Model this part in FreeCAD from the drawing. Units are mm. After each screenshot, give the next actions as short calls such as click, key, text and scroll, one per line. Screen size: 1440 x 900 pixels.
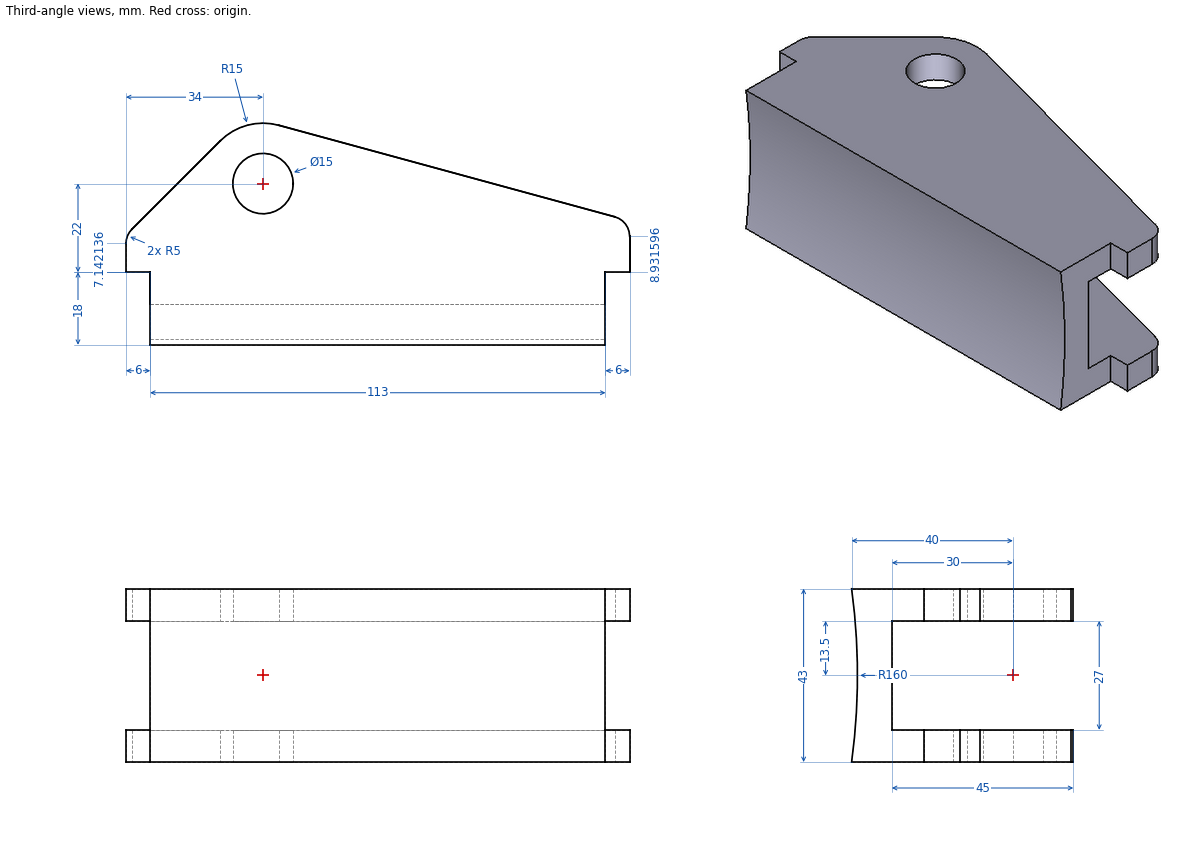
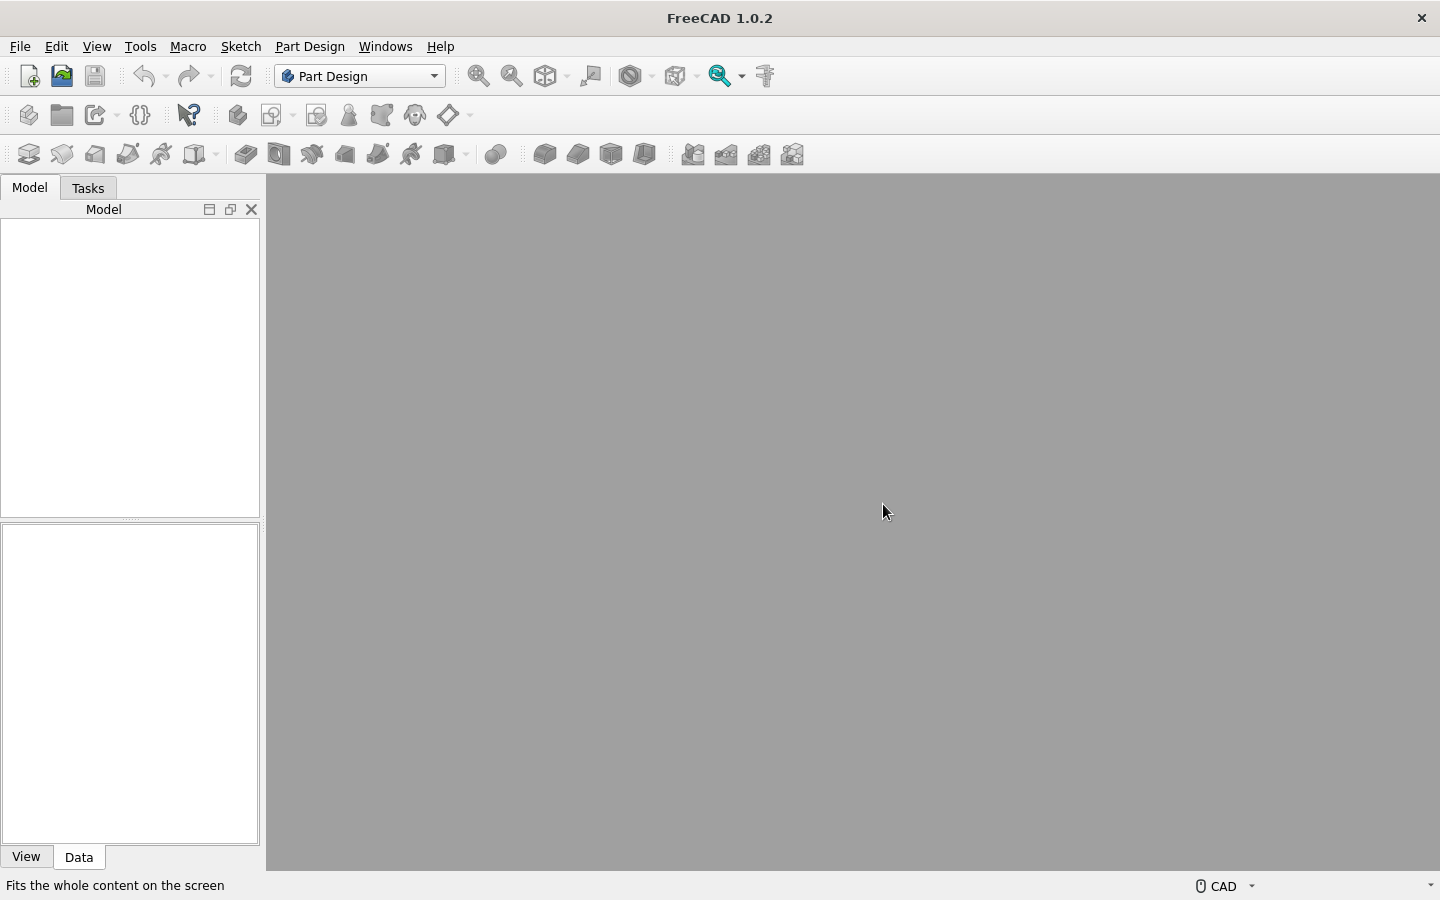
click(29, 76)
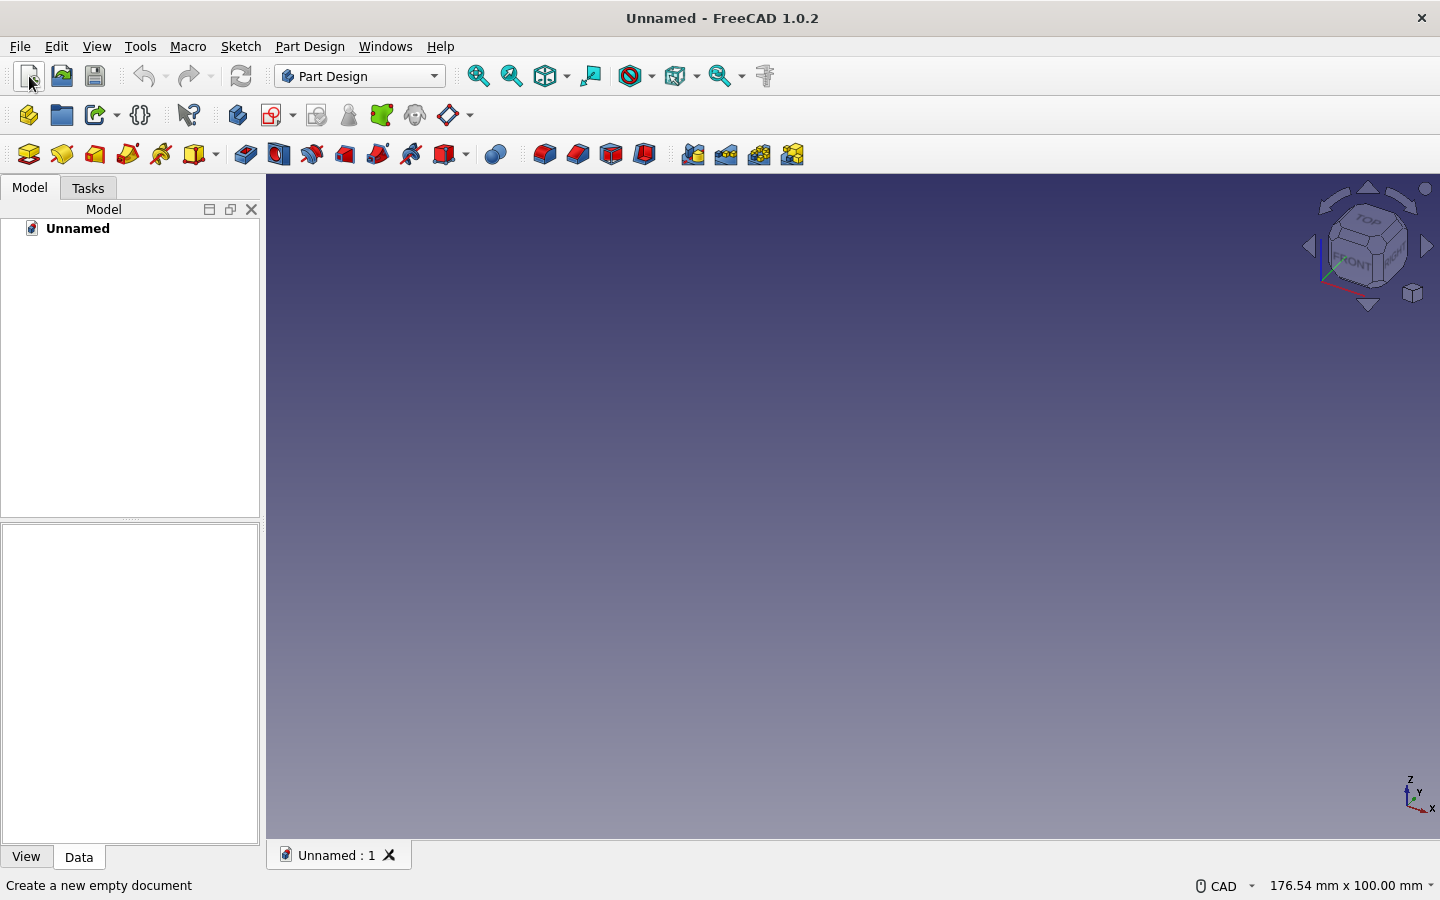
click(270, 116)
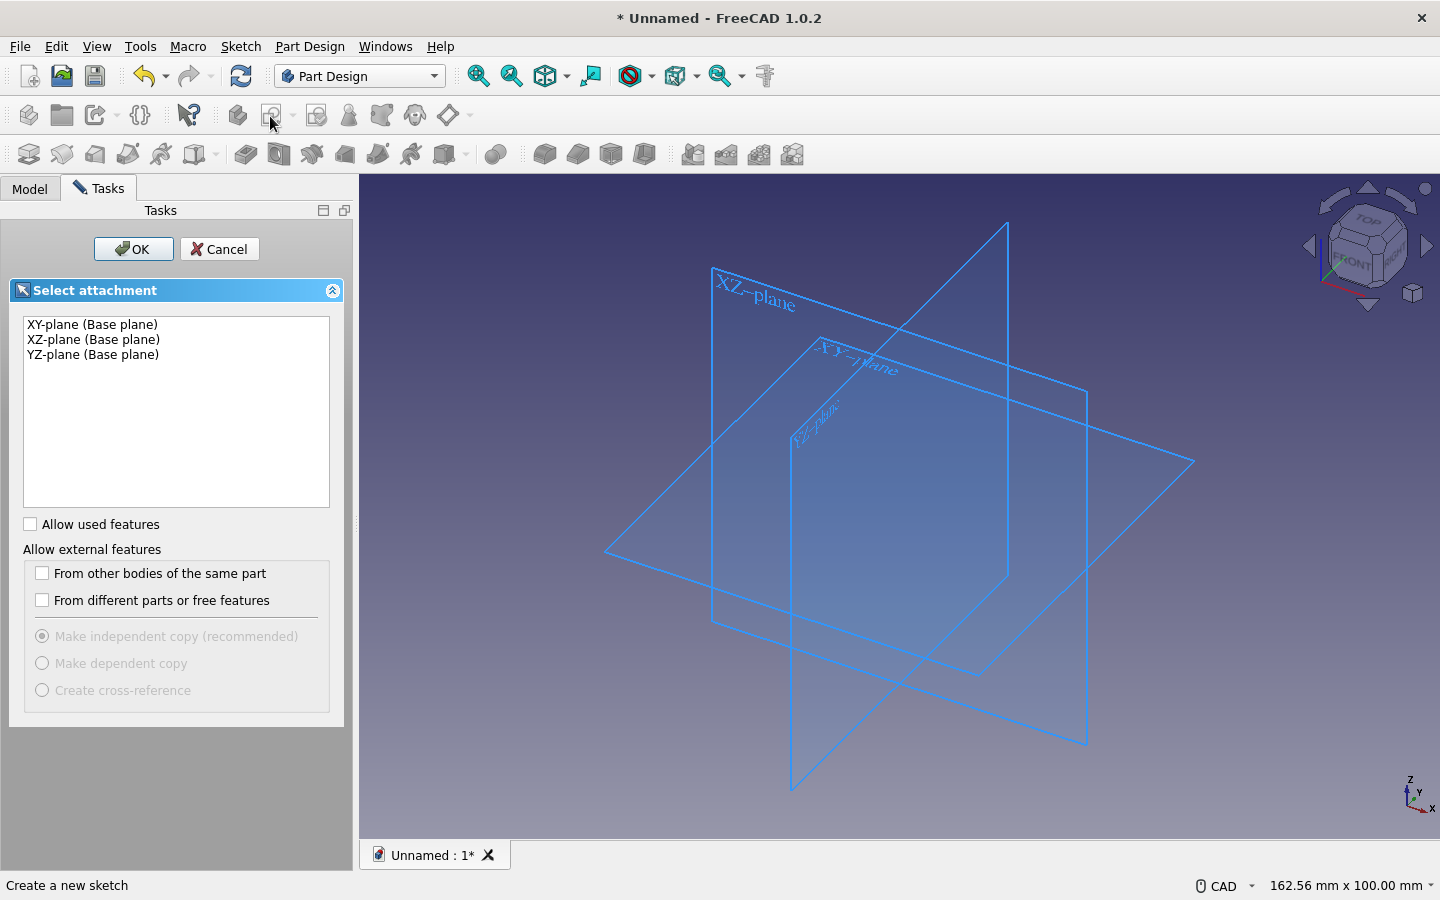
click(84, 324)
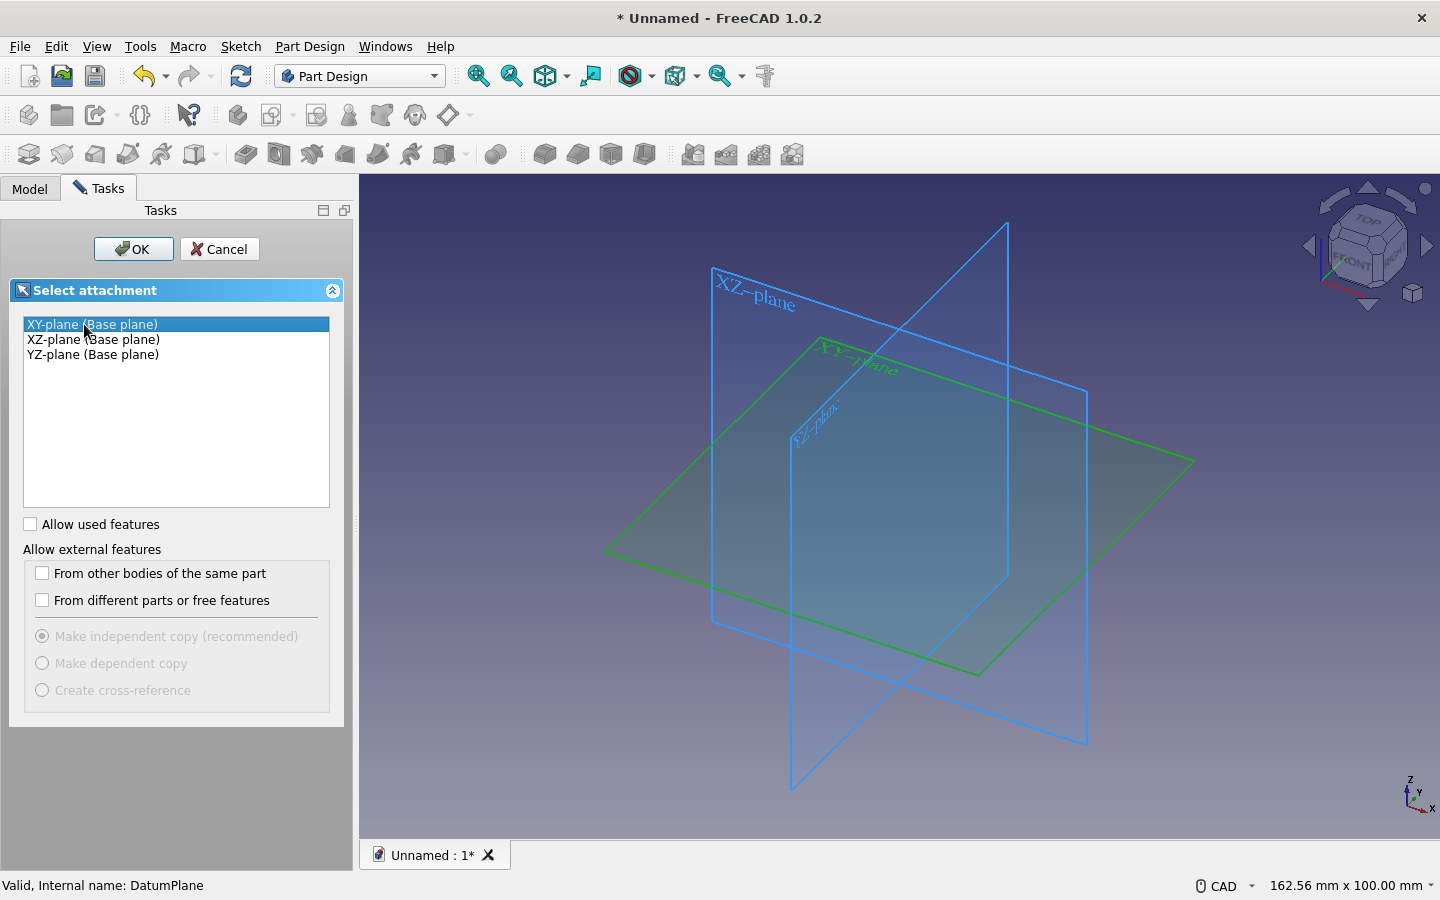
click(134, 249)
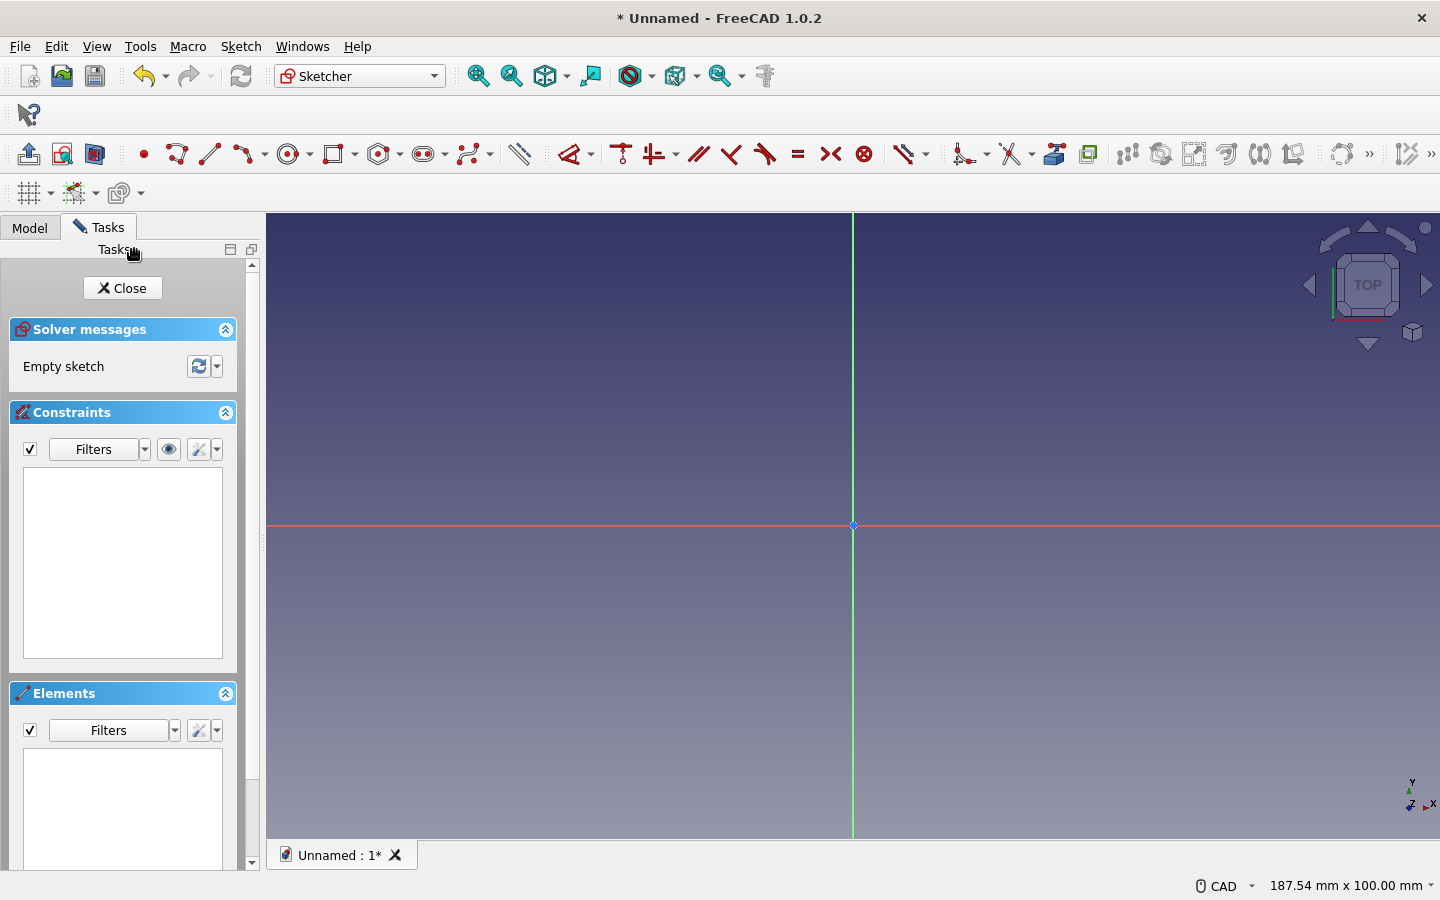
scroll(294, 241, down, 1)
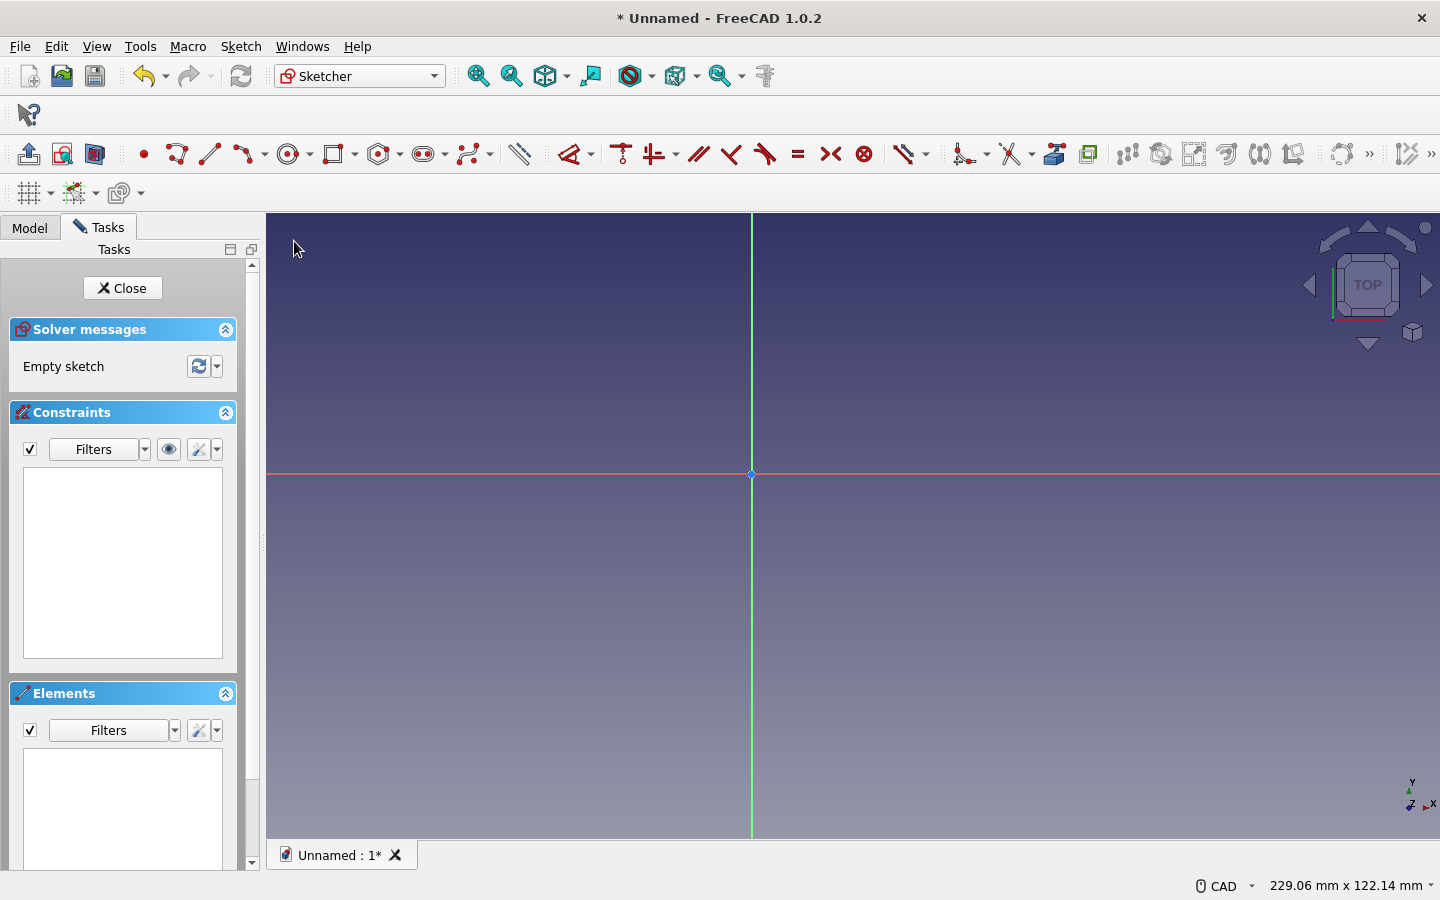
click(177, 154)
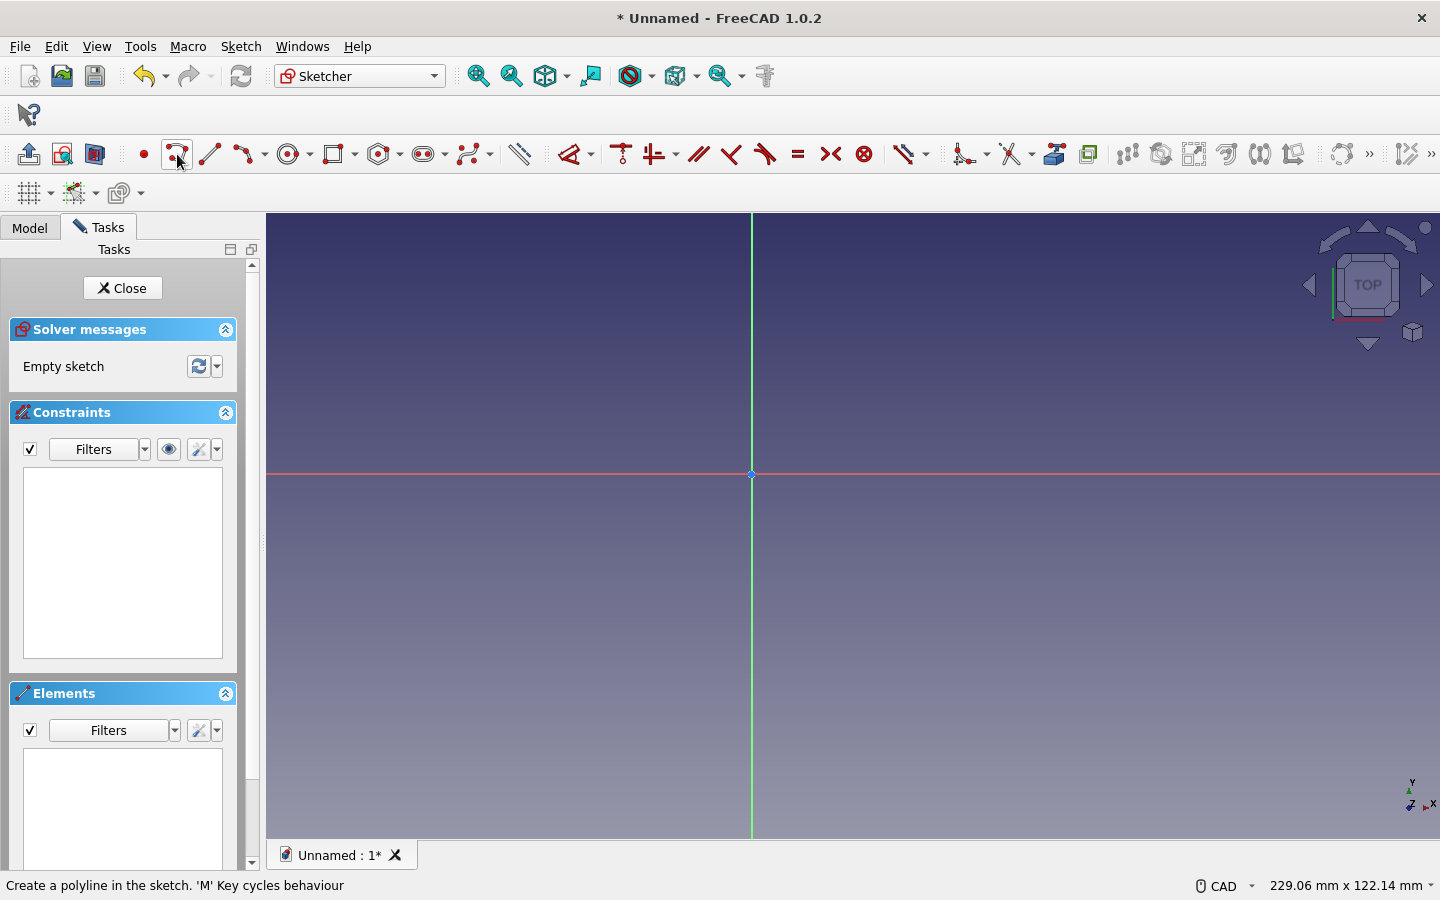
click(577, 550)
click(577, 587)
click(608, 587)
click(608, 679)
click(1187, 679)
click(1187, 587)
click(1218, 587)
click(1218, 541)
right_click(1218, 541)